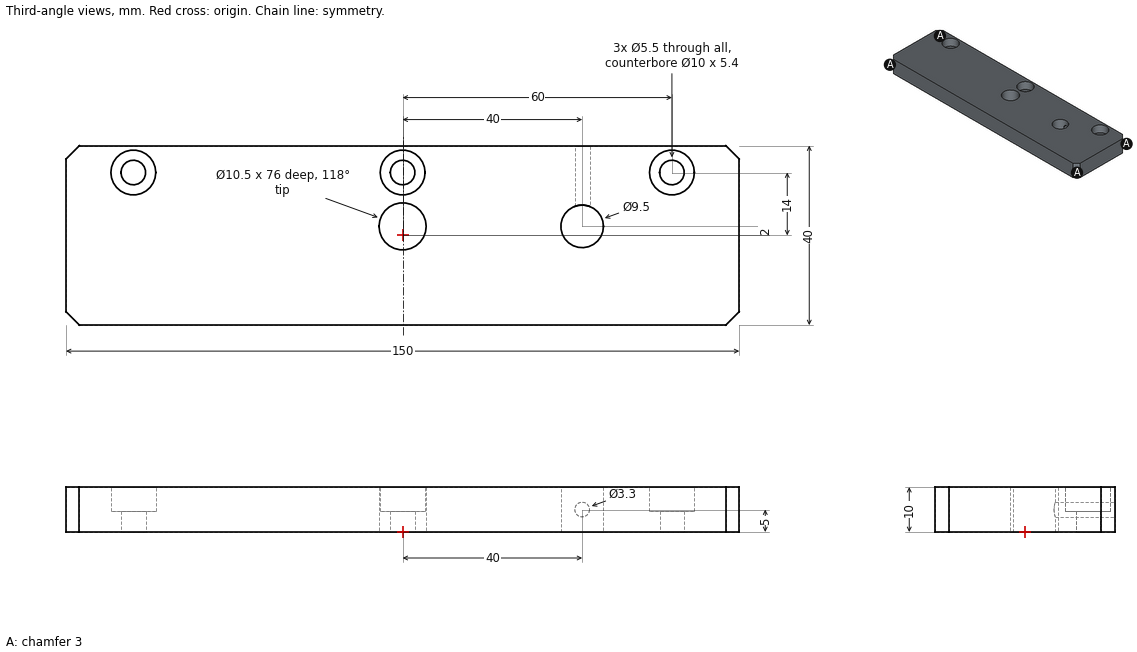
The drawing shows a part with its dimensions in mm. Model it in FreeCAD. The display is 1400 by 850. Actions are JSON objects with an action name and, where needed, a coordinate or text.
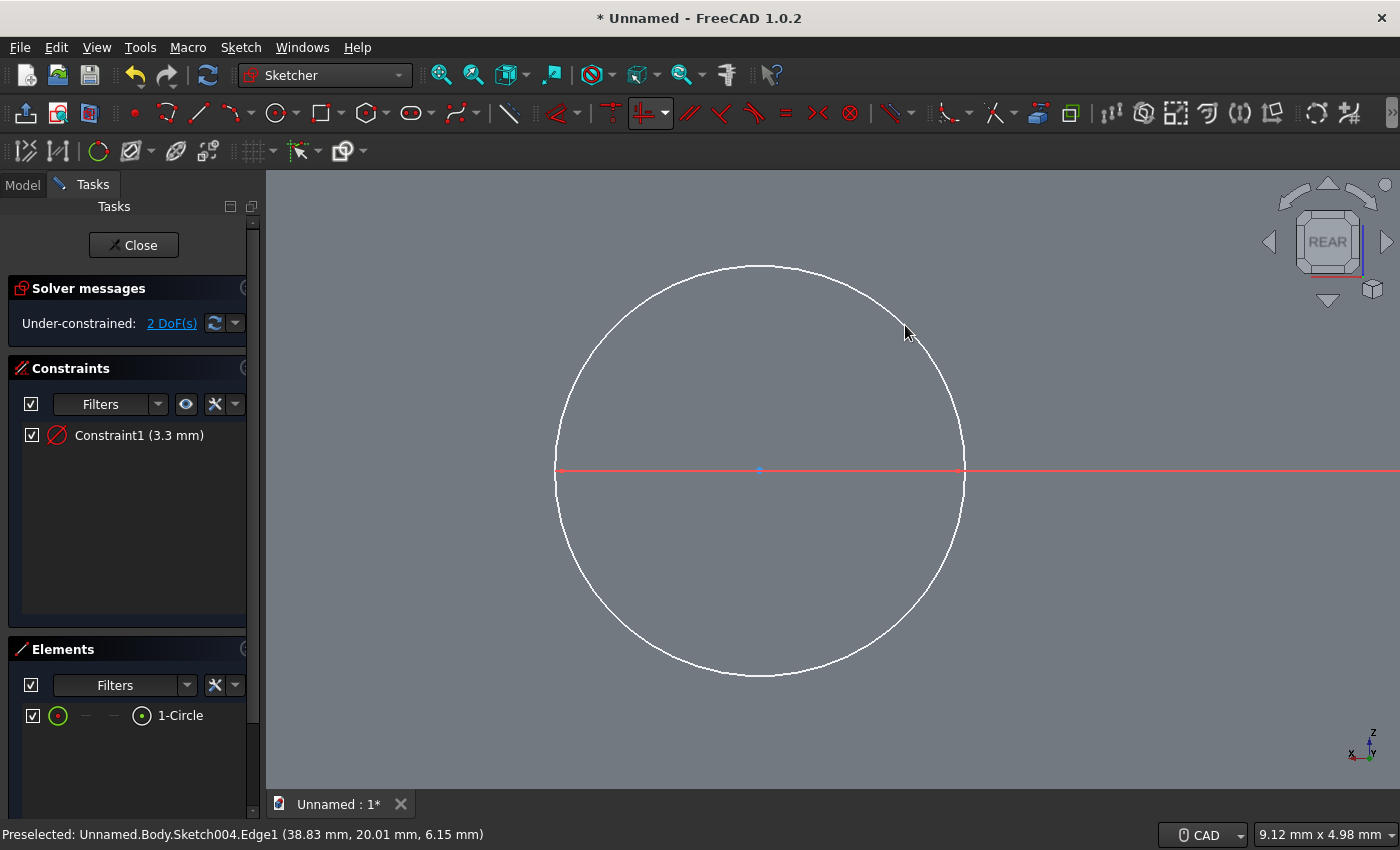
{"action": "key", "text": "d"}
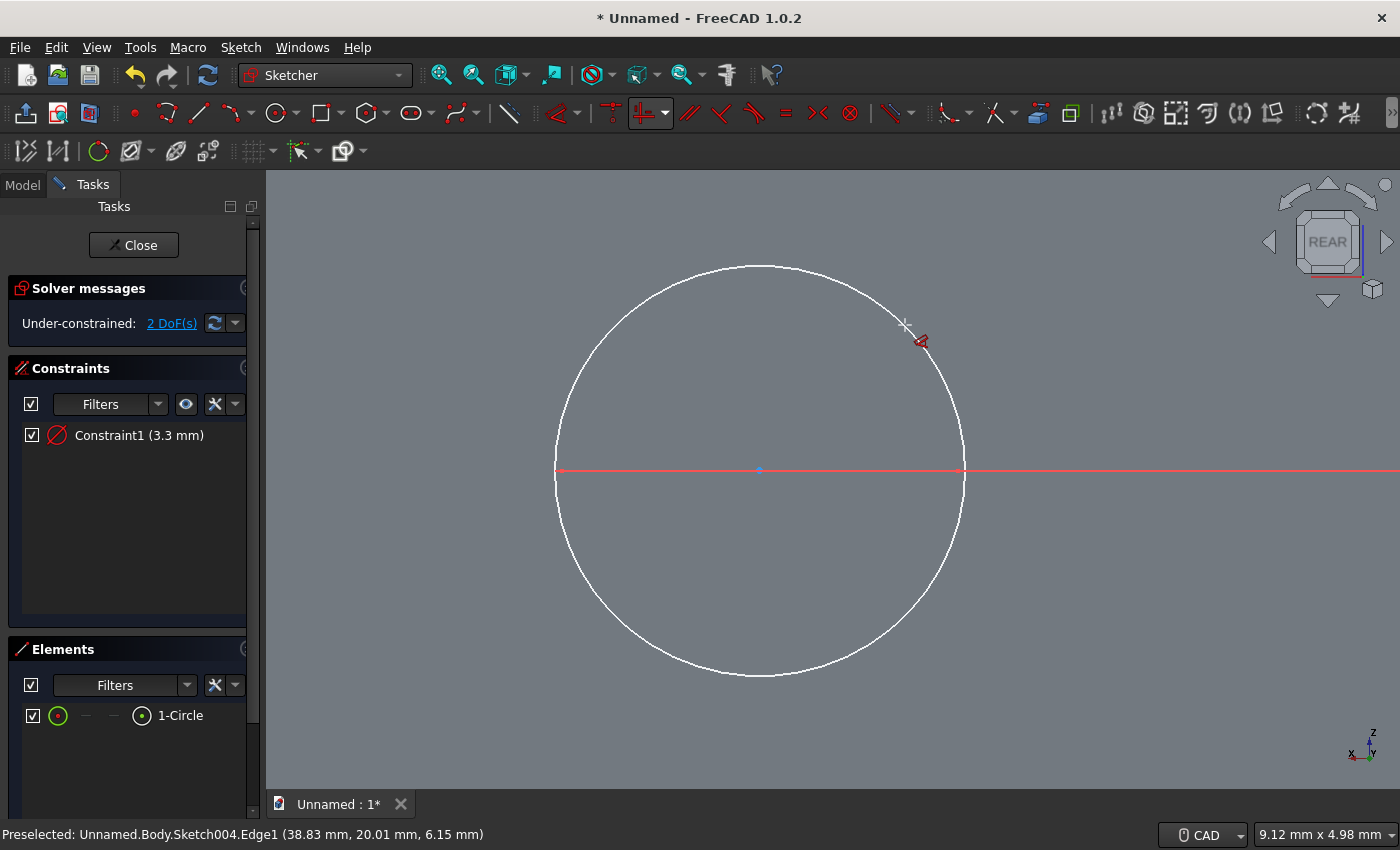
{"action": "left_click", "coordinate": [760, 471]}
{"action": "left_click", "coordinate": [726, 616]}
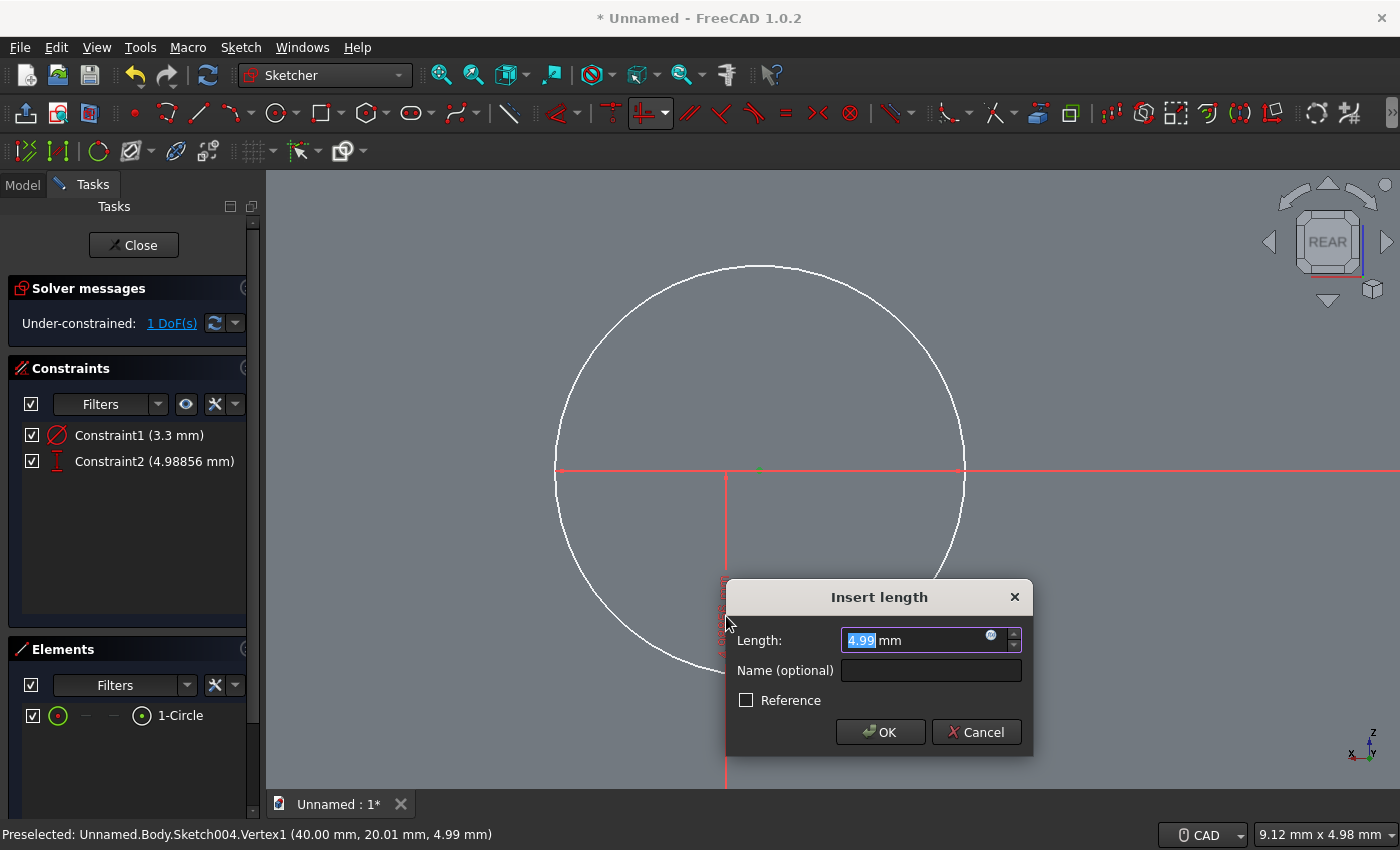
{"action": "type", "text": "5"}
{"action": "key", "text": "Return"}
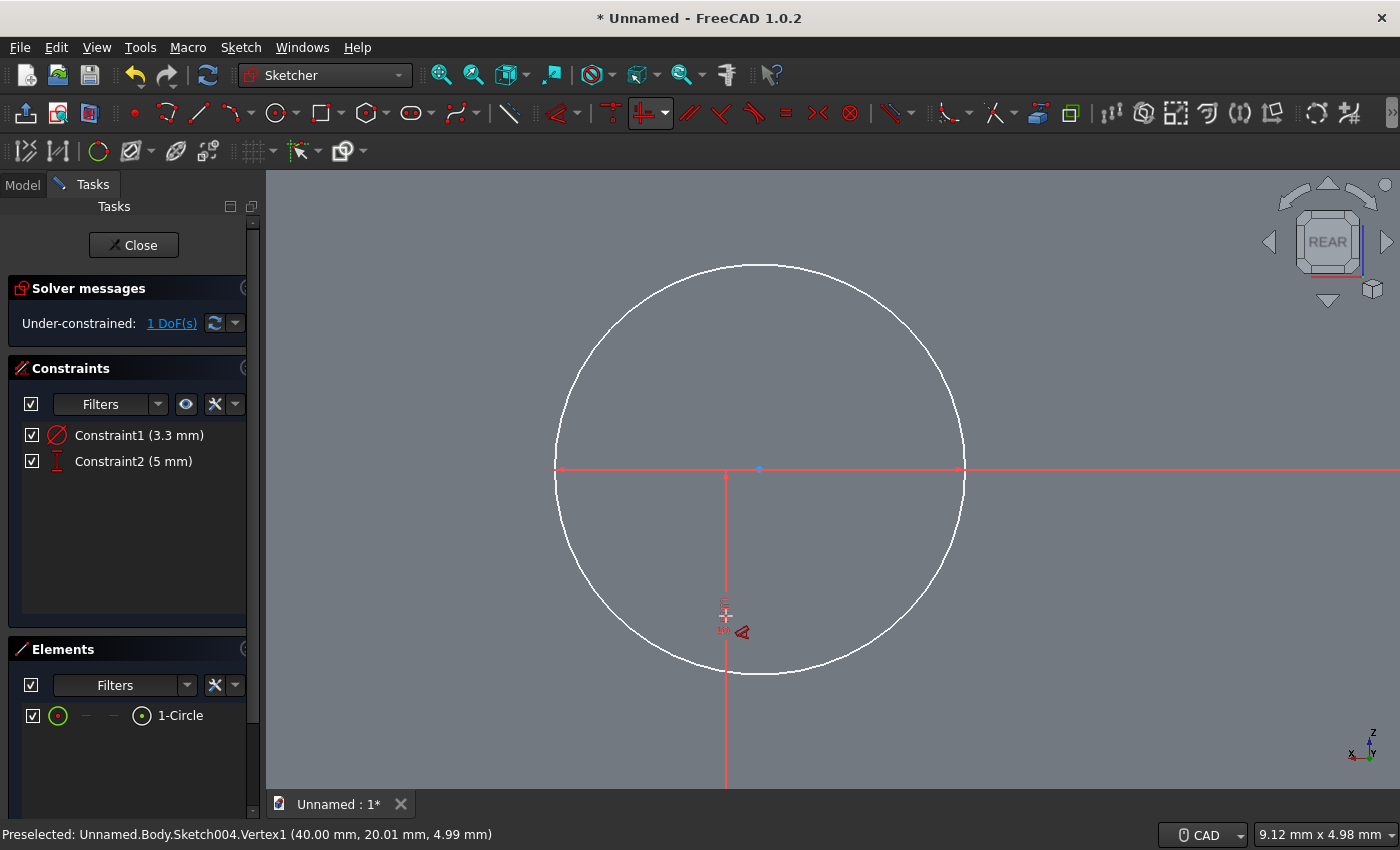
{"action": "left_click", "coordinate": [760, 470]}
{"action": "left_click", "coordinate": [997, 436]}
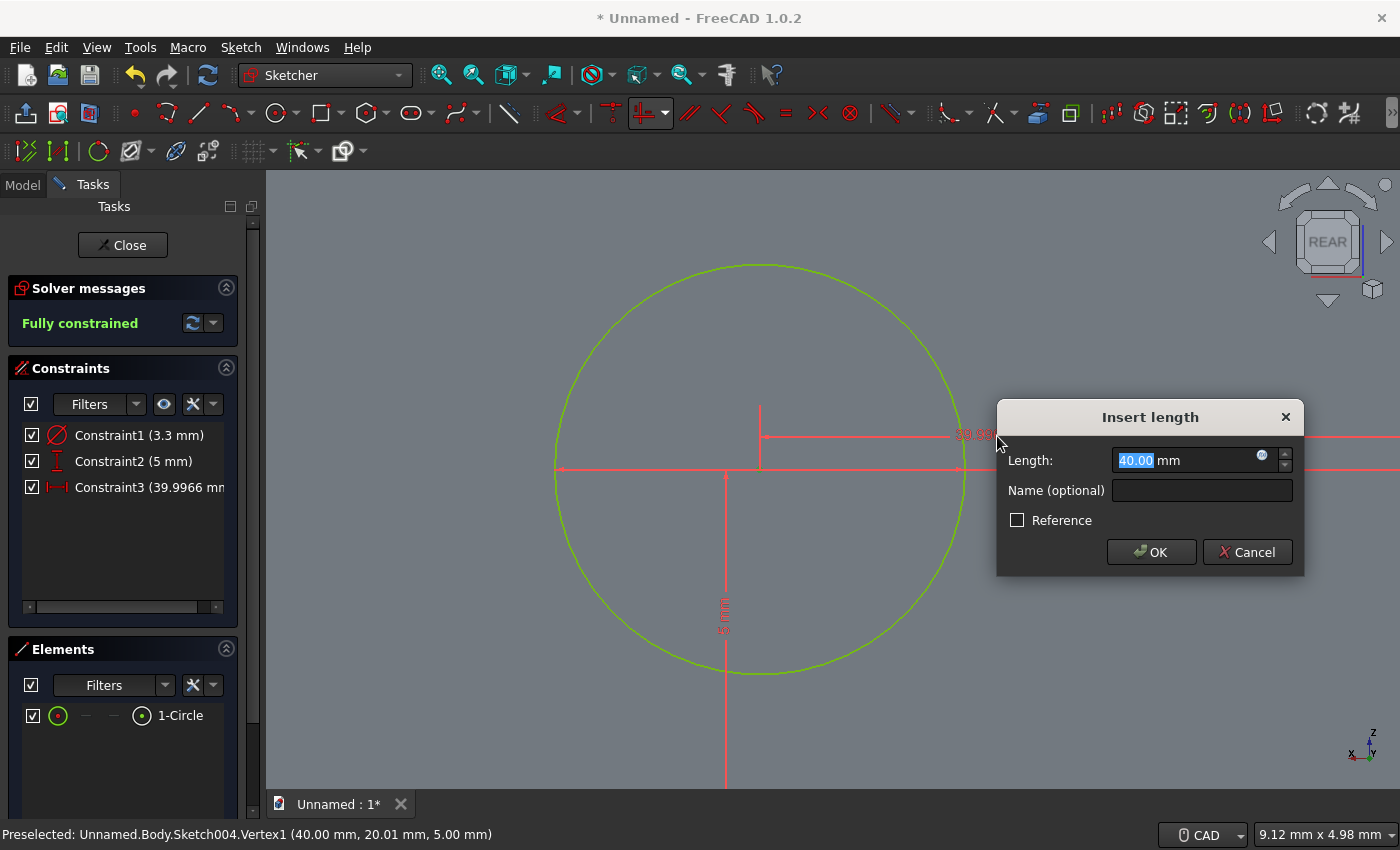
{"action": "type", "text": "40"}
{"action": "key", "text": "Return"}
{"action": "key", "text": "Escape"}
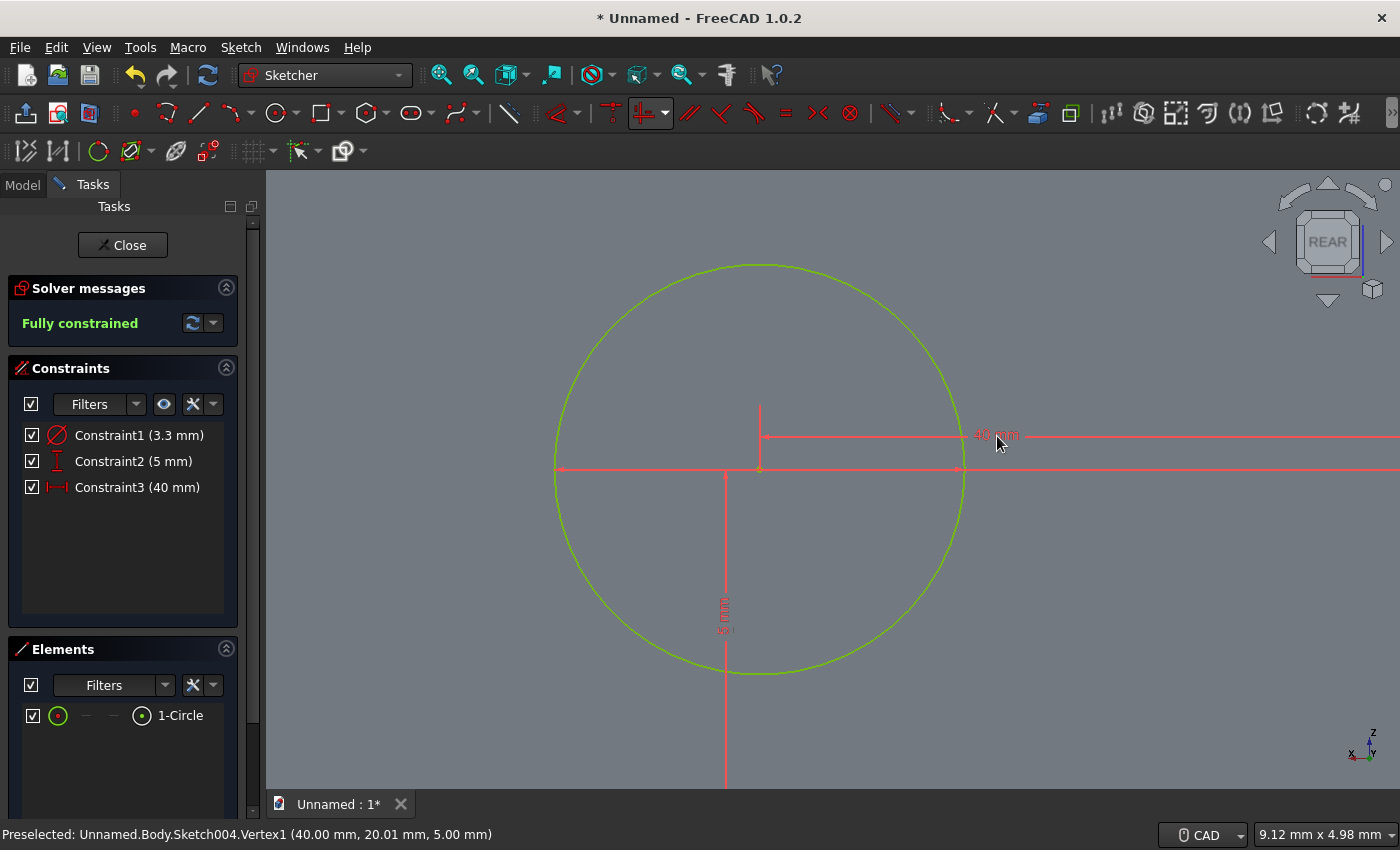
{"action": "left_click", "coordinate": [123, 245]}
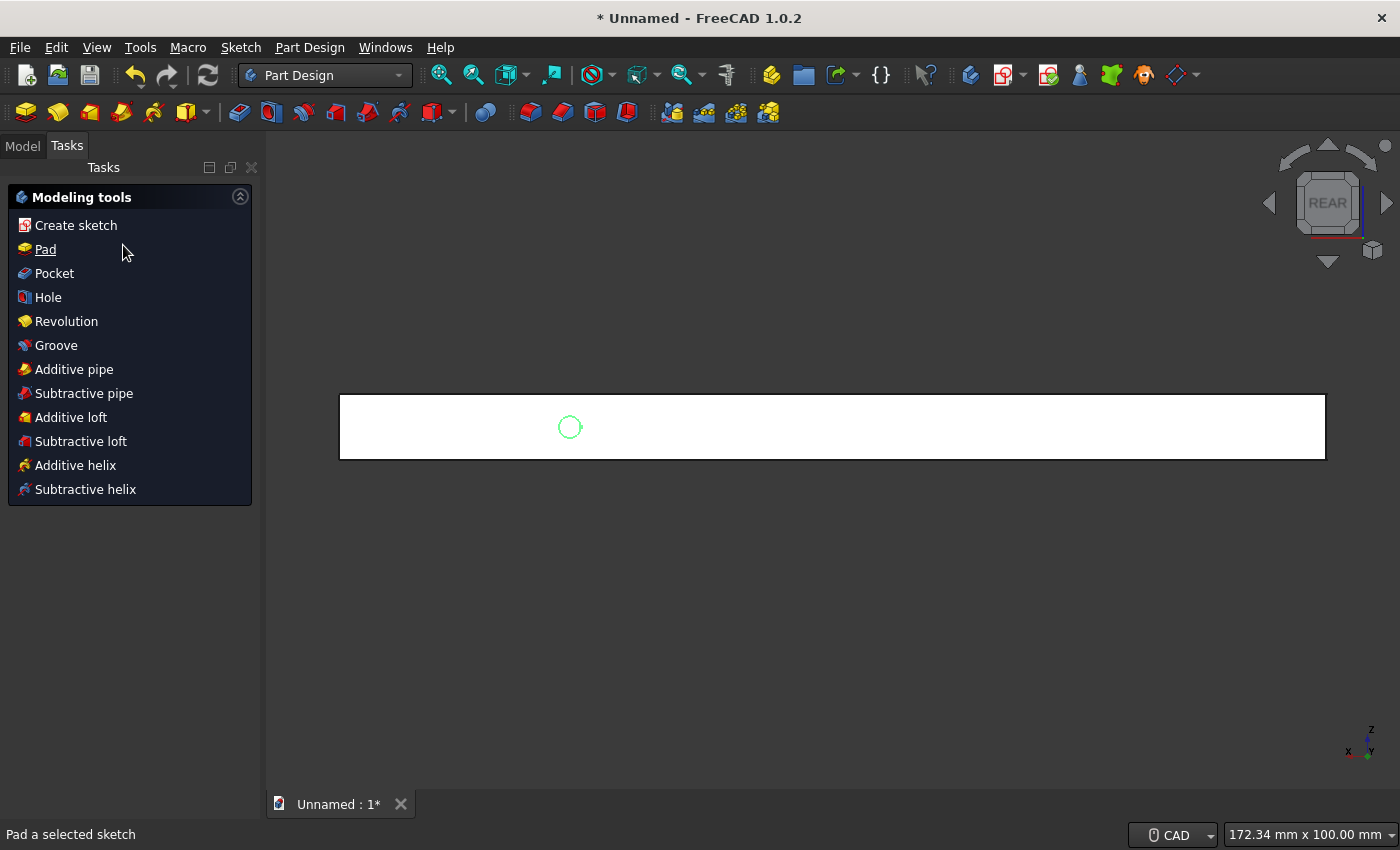
{"action": "left_click", "coordinate": [240, 112]}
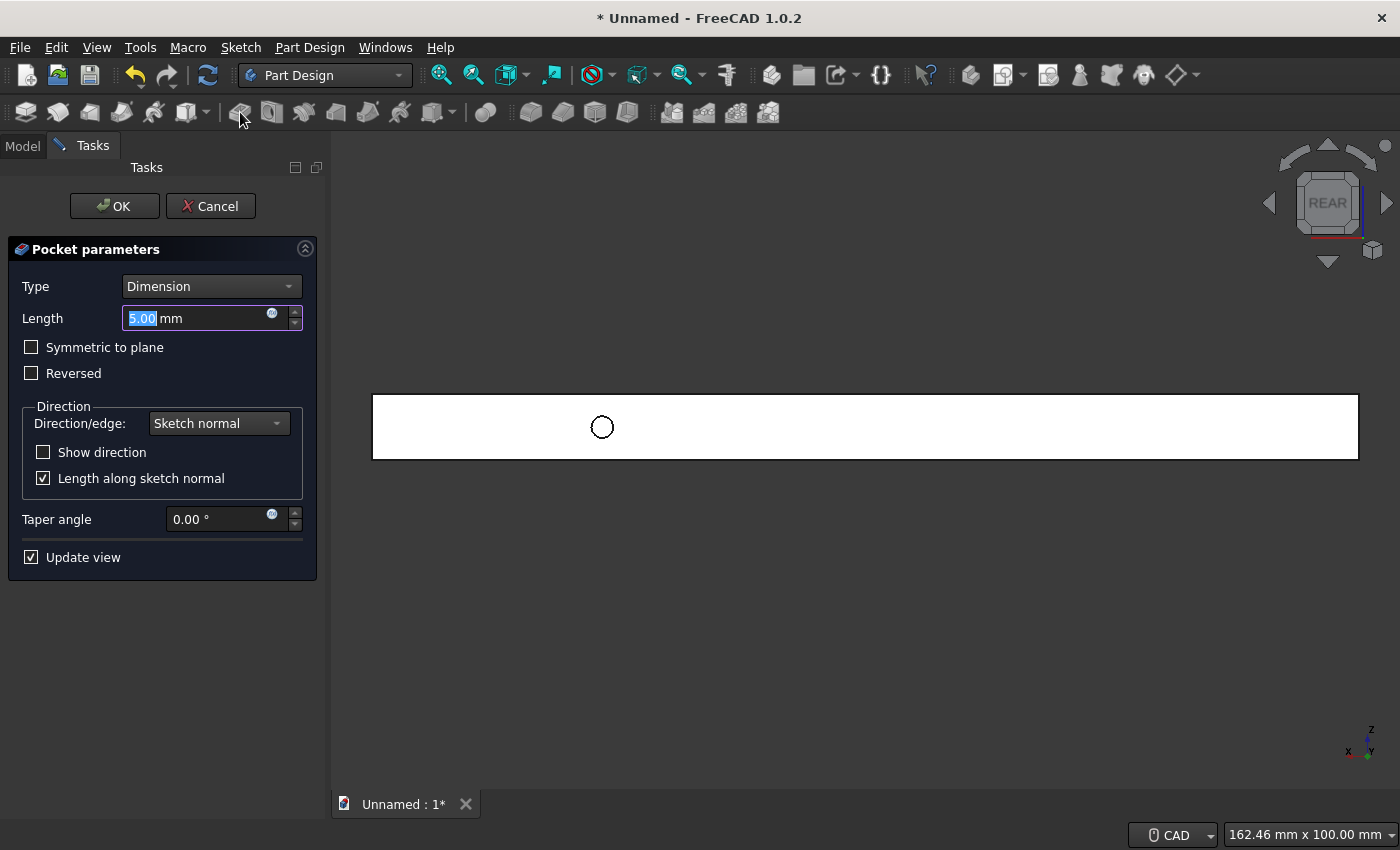
{"action": "left_click", "coordinate": [212, 286]}